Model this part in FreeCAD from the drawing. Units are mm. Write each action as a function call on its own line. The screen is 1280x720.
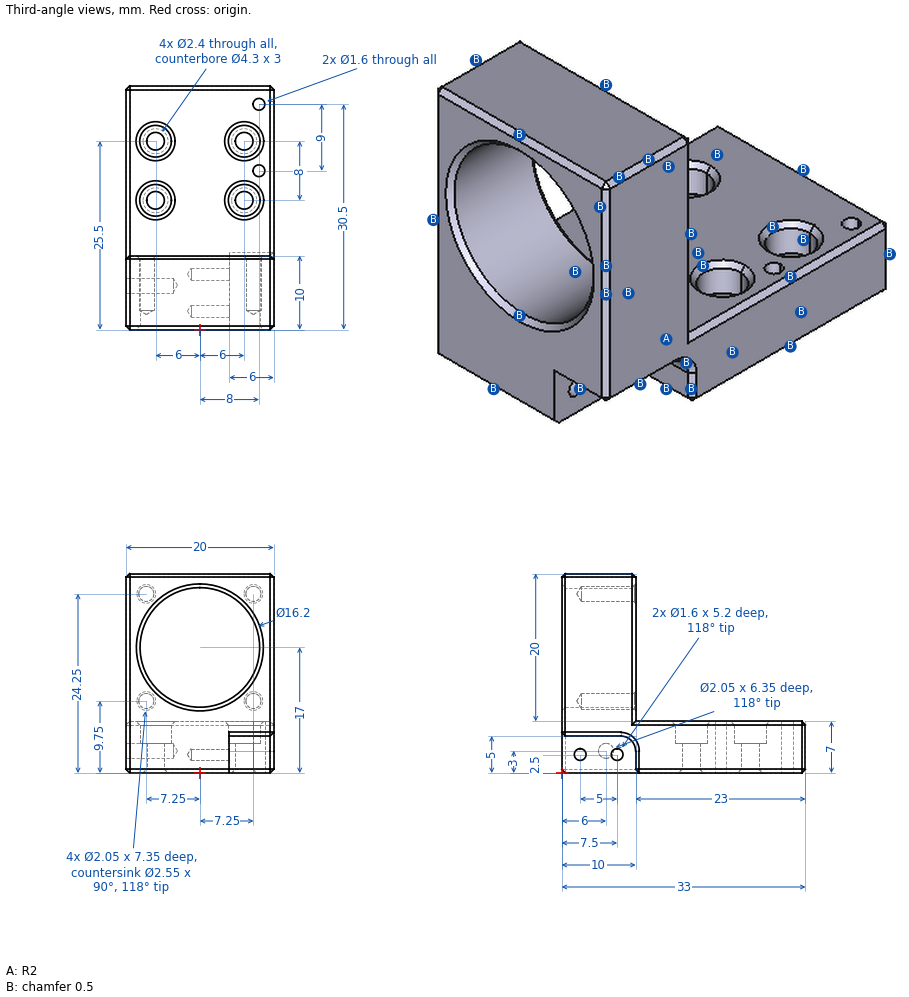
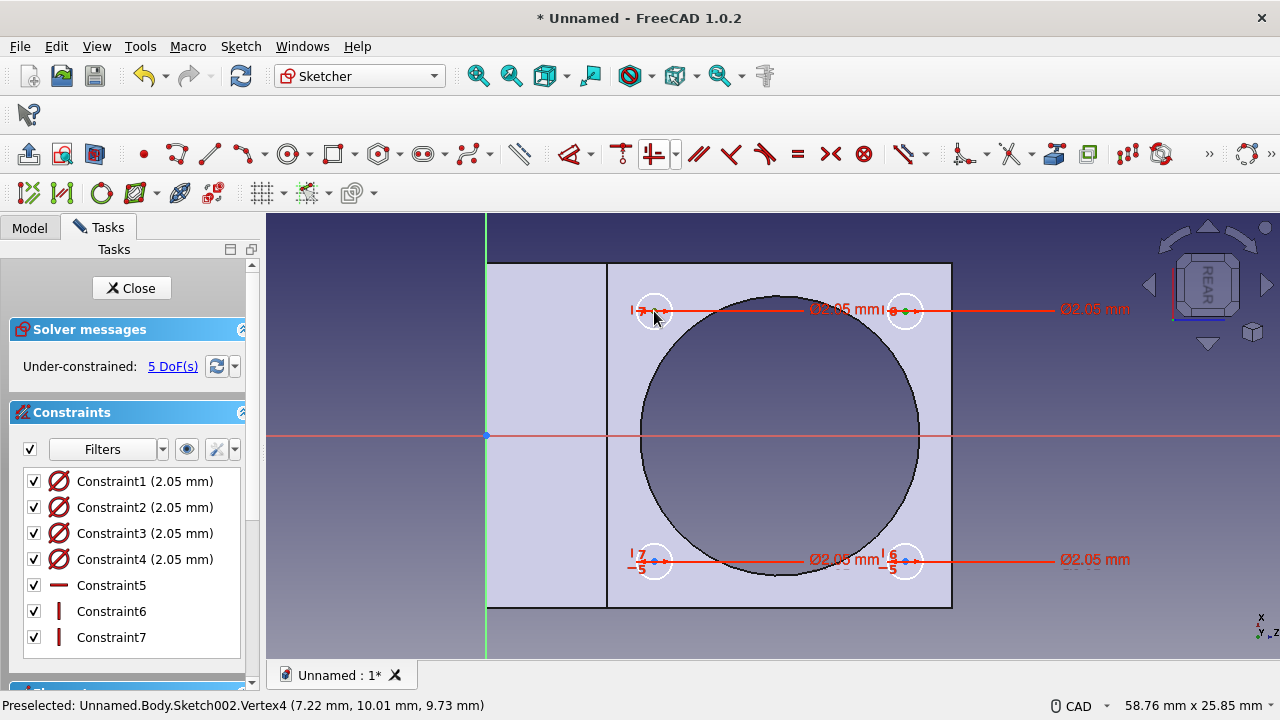
key(h)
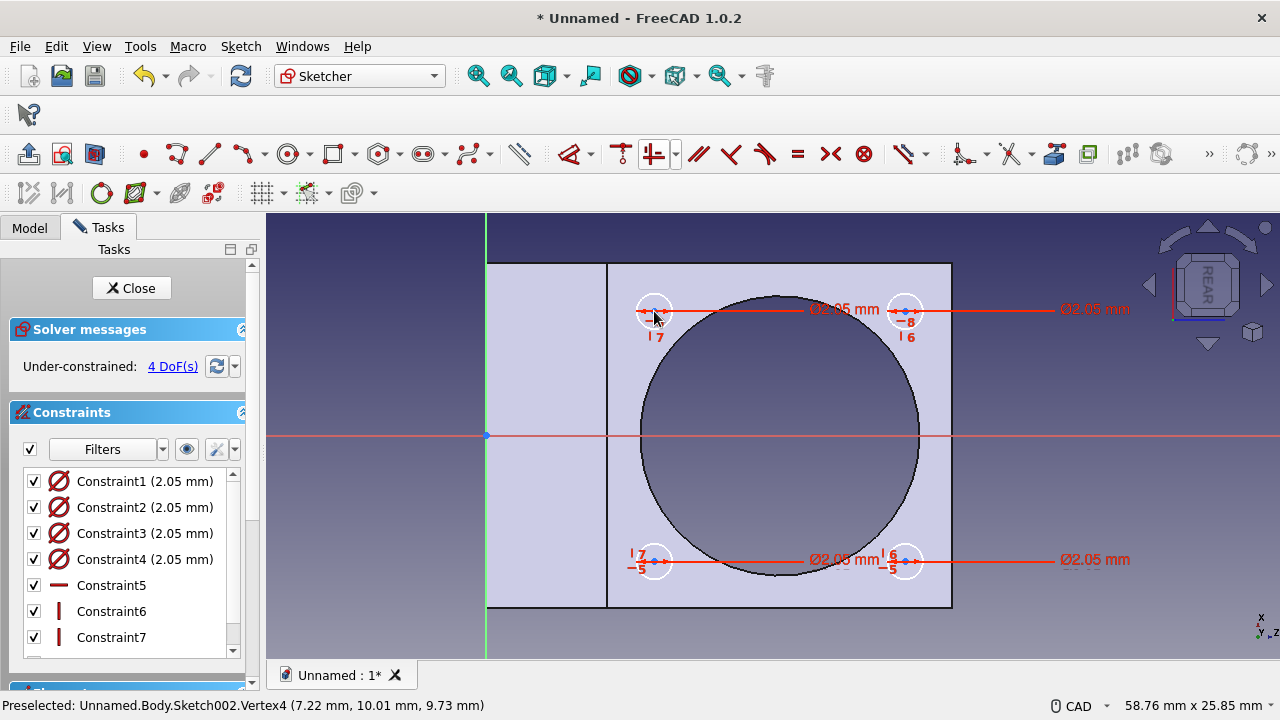
click(568, 154)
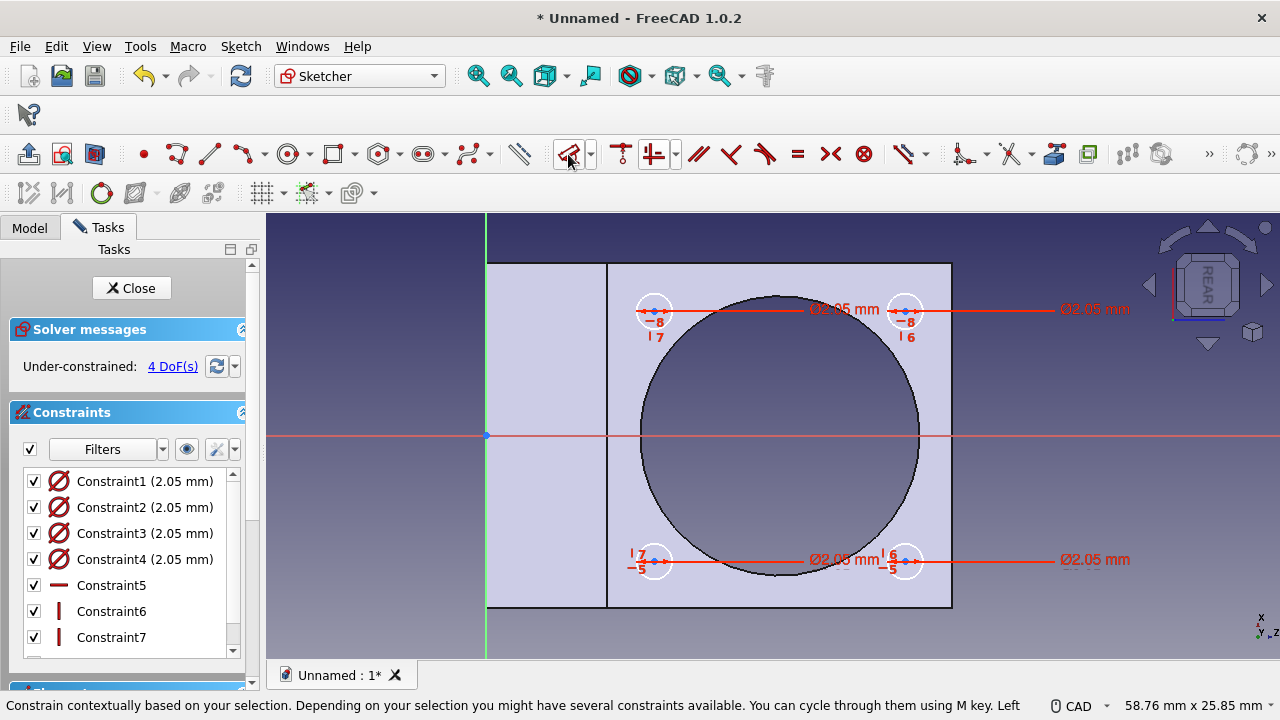
click(654, 562)
click(570, 596)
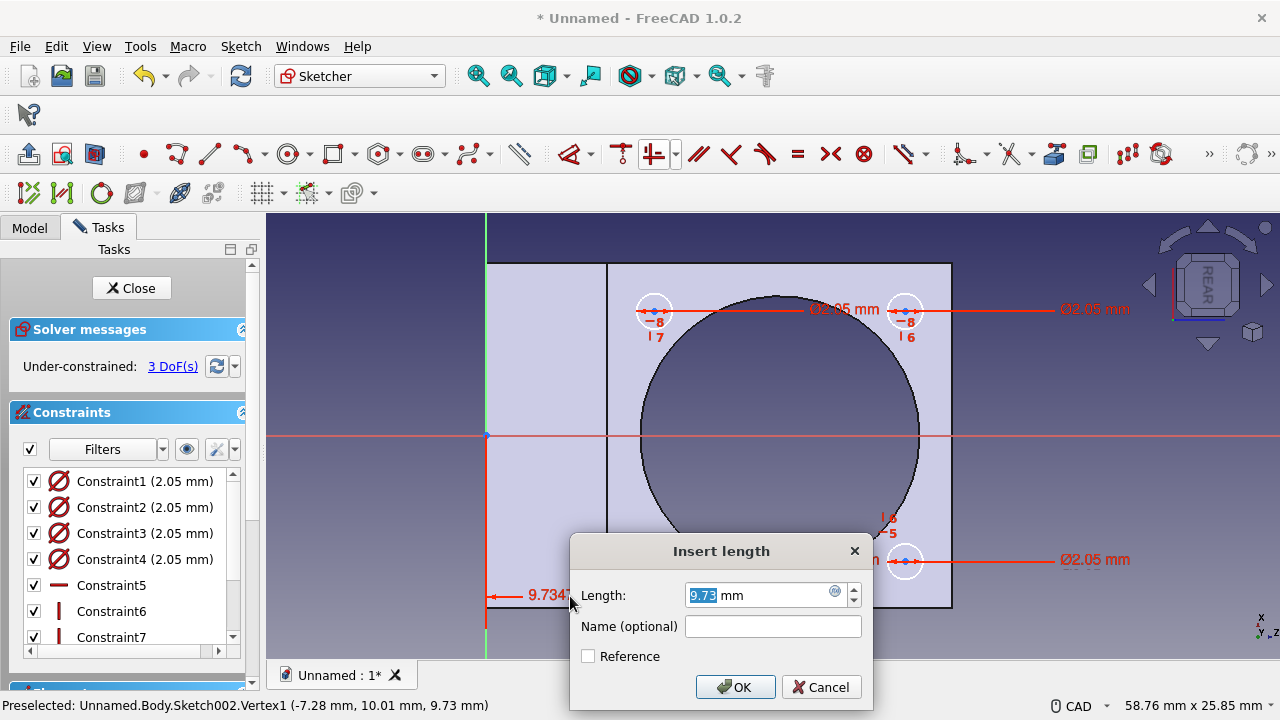
text(9.75)
key(Return)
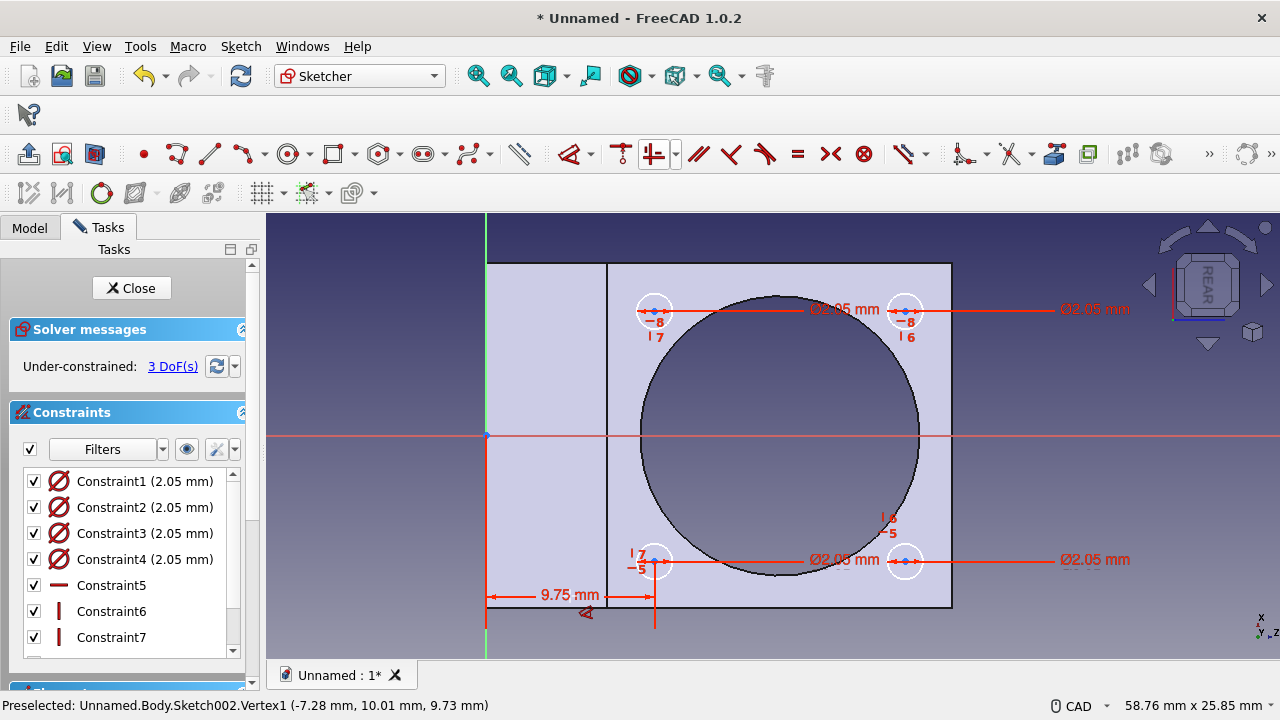
click(655, 562)
click(452, 499)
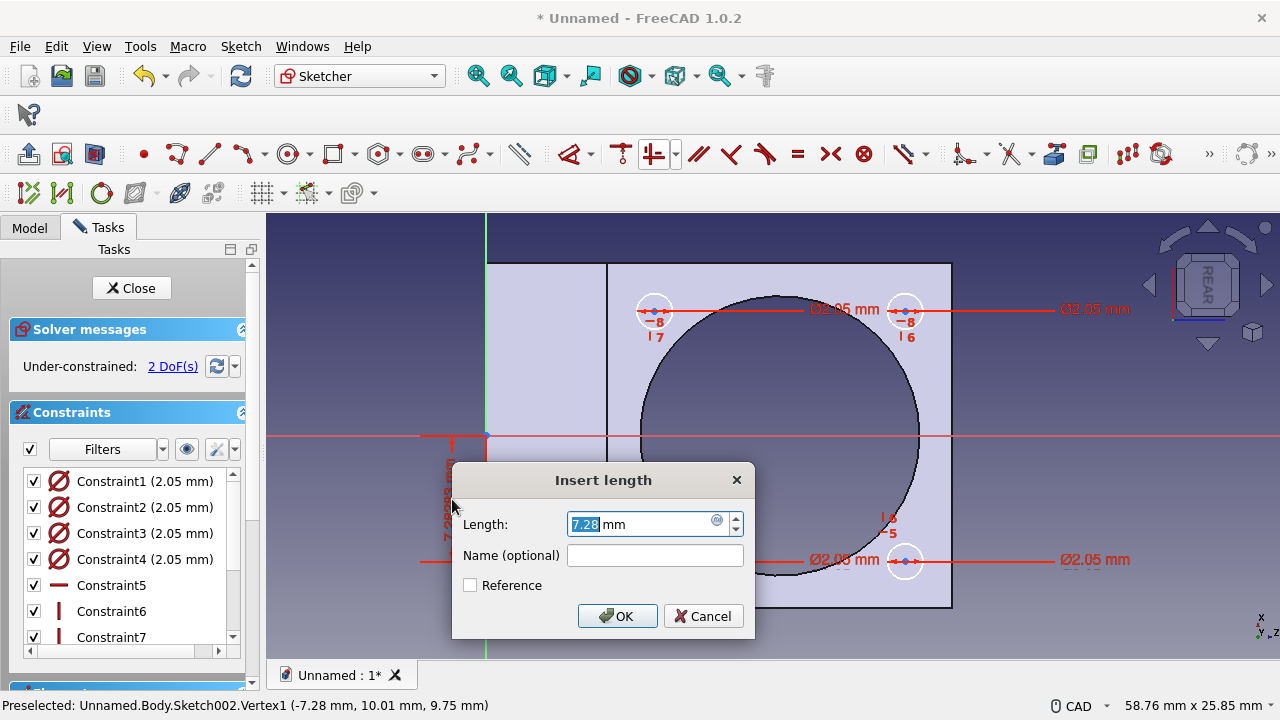
text(7.25)
key(Return)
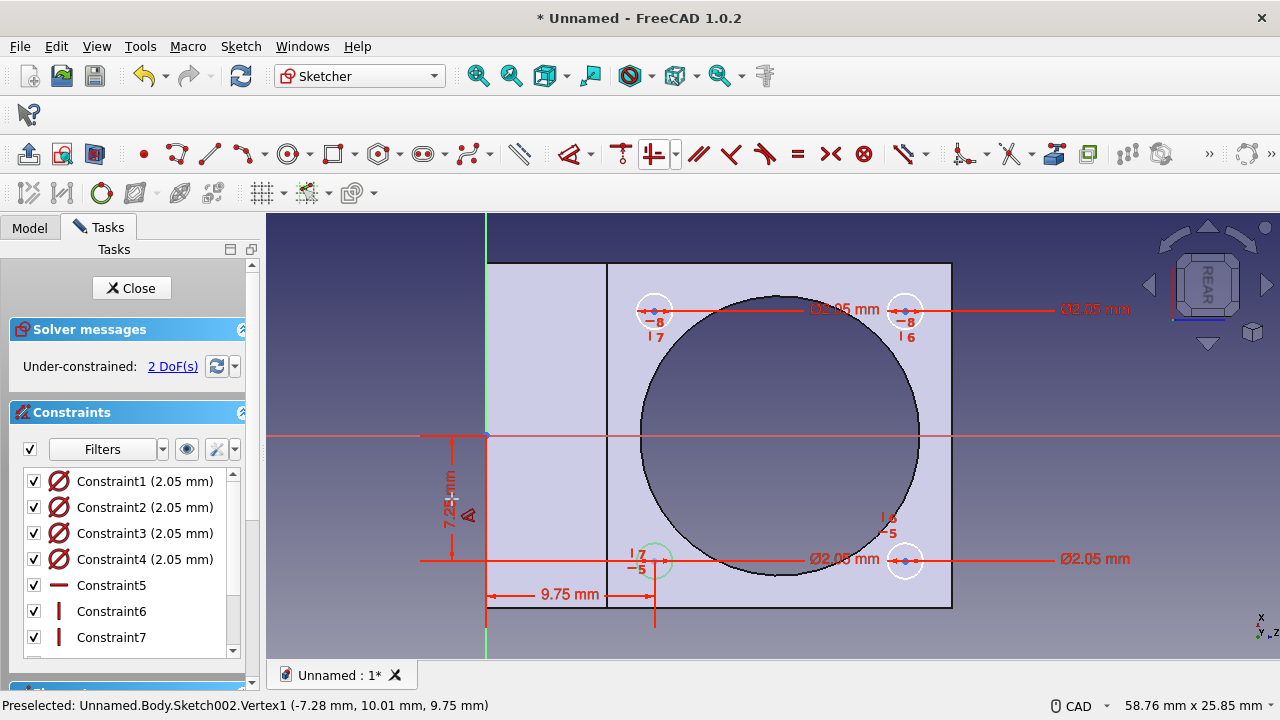
click(905, 311)
click(452, 374)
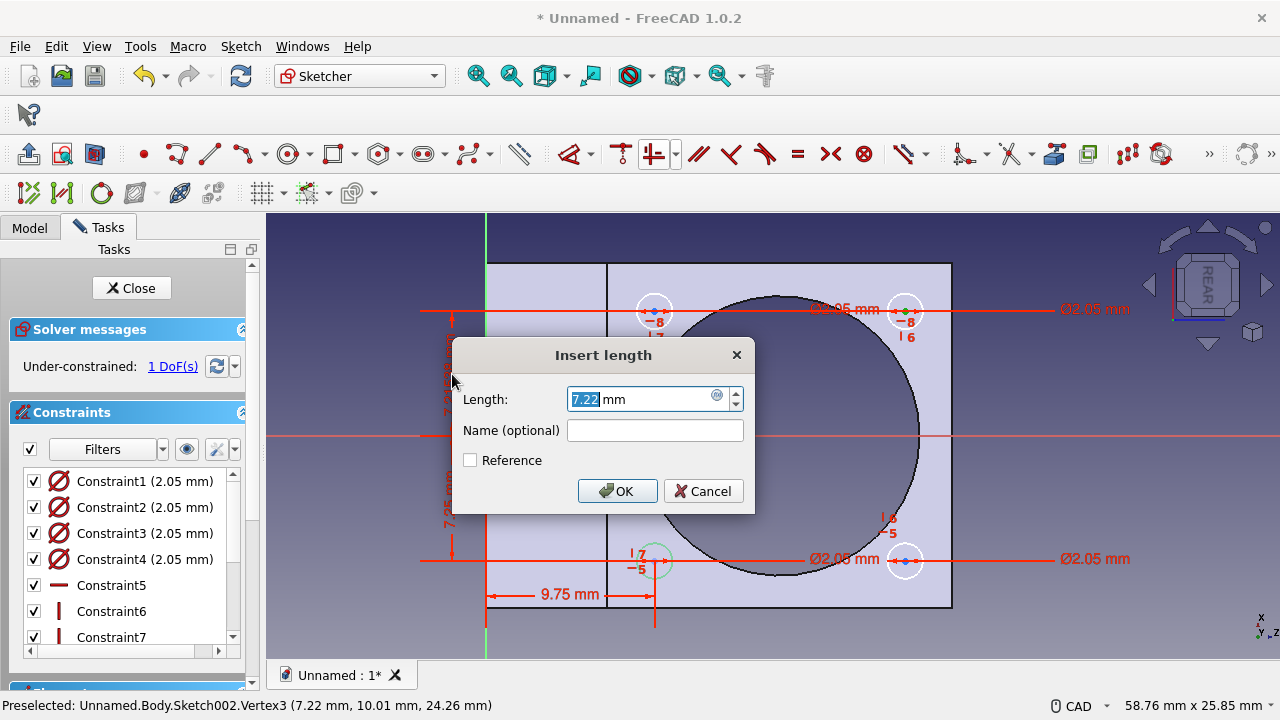
text(7.25)
key(Return)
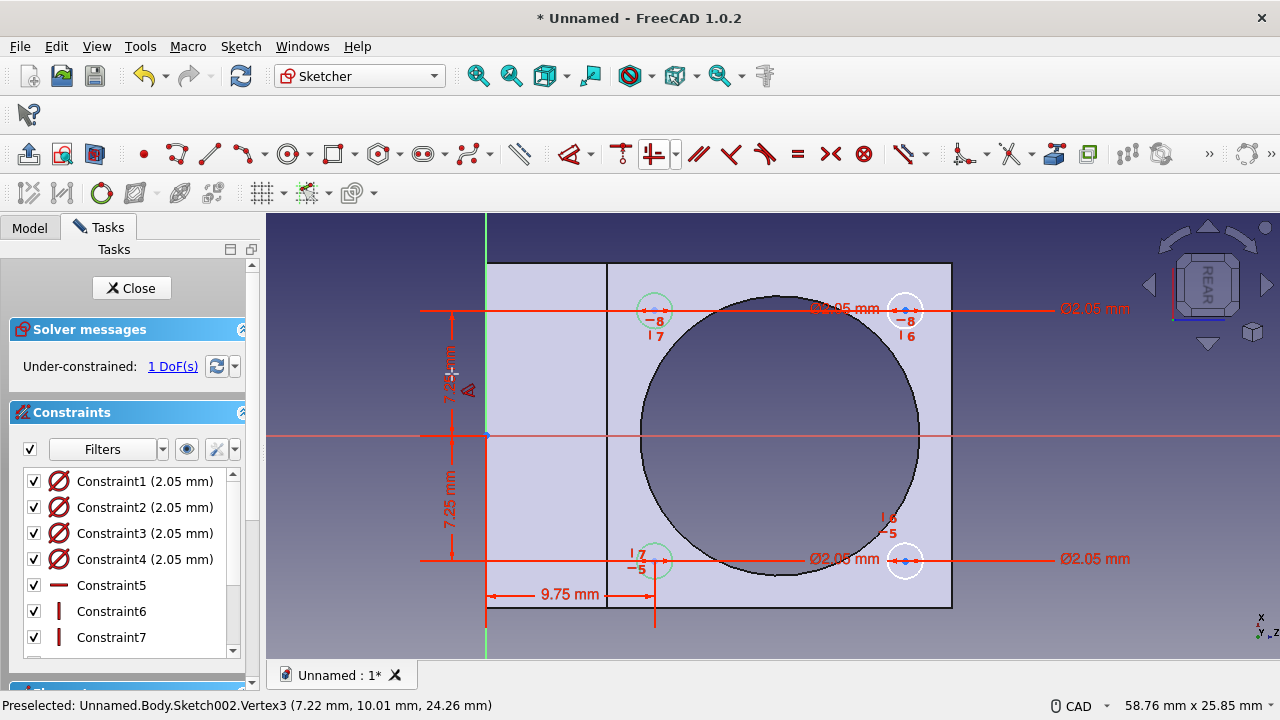
click(905, 561)
click(696, 595)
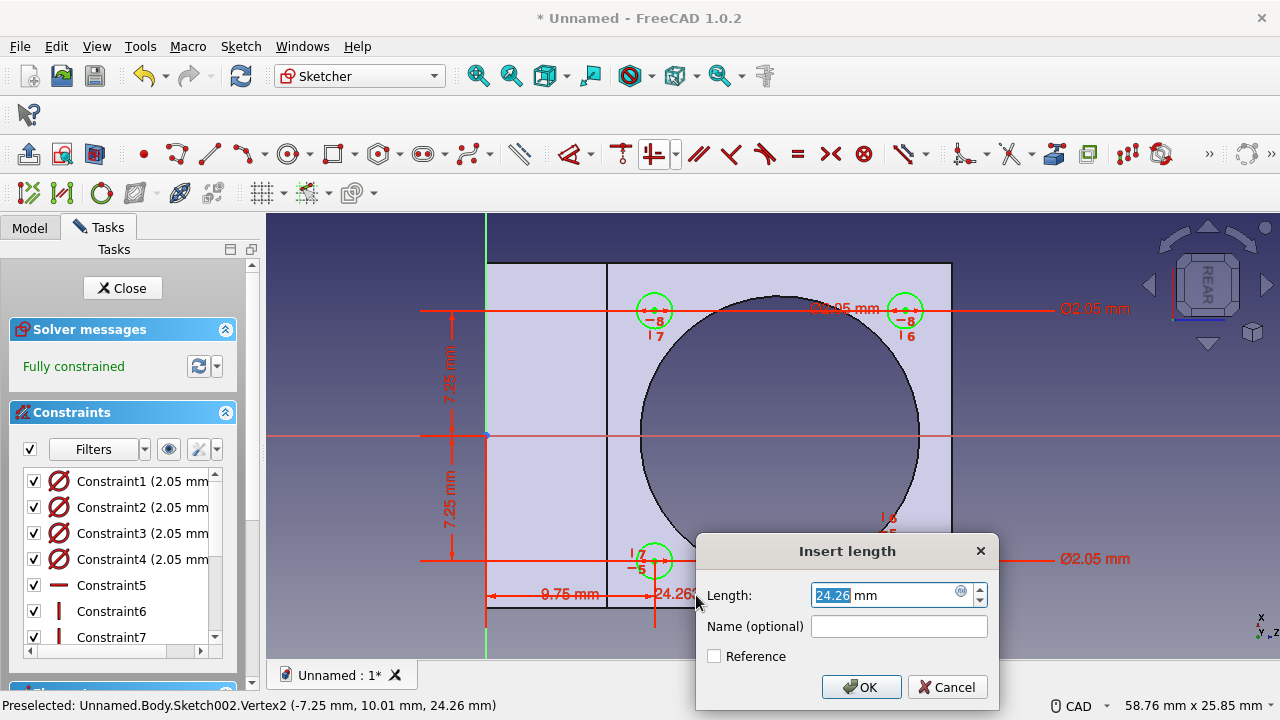
text(24.25)
key(Return)
key(Escape)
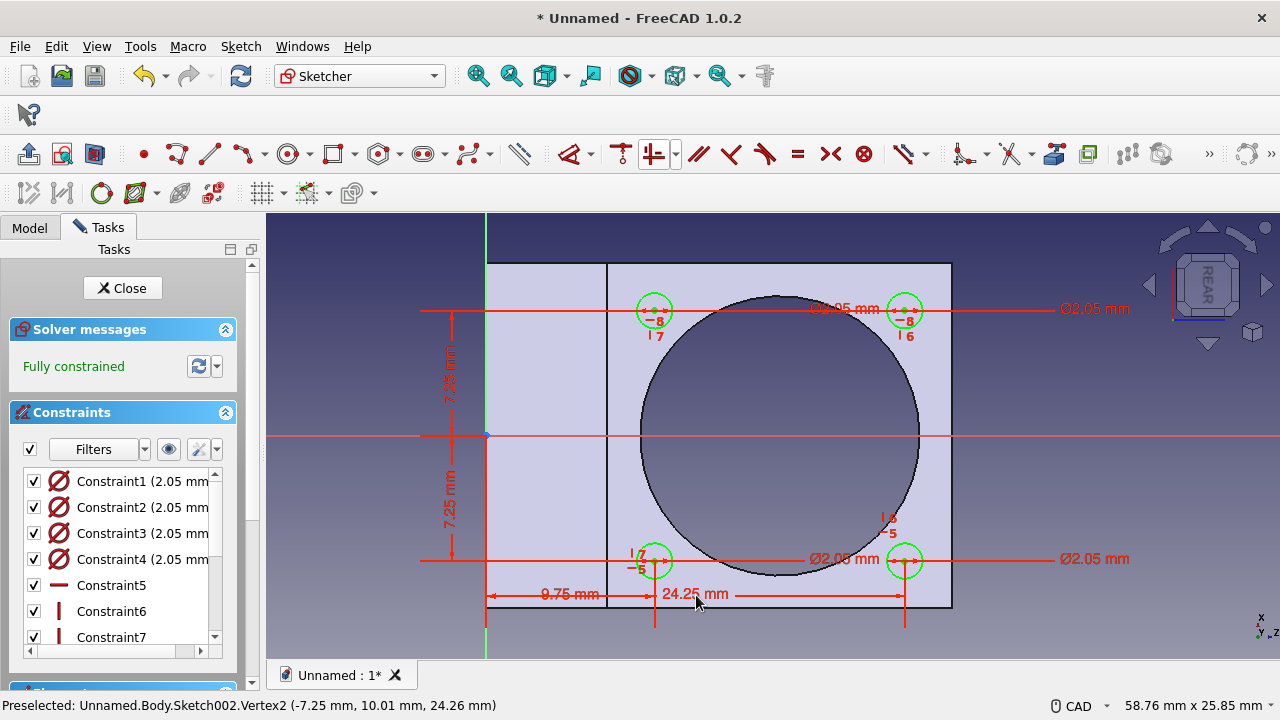
click(123, 288)